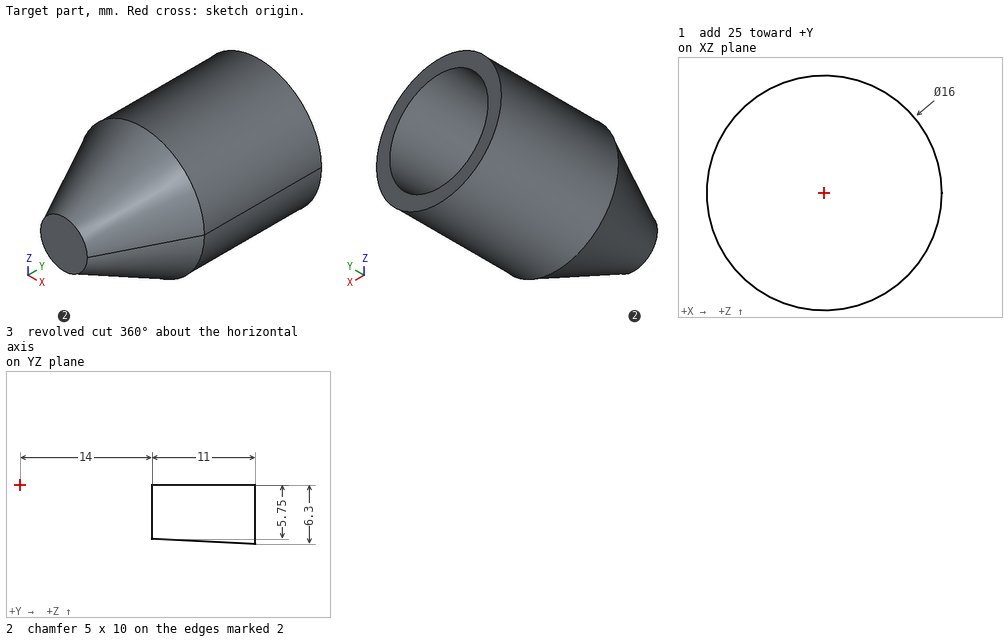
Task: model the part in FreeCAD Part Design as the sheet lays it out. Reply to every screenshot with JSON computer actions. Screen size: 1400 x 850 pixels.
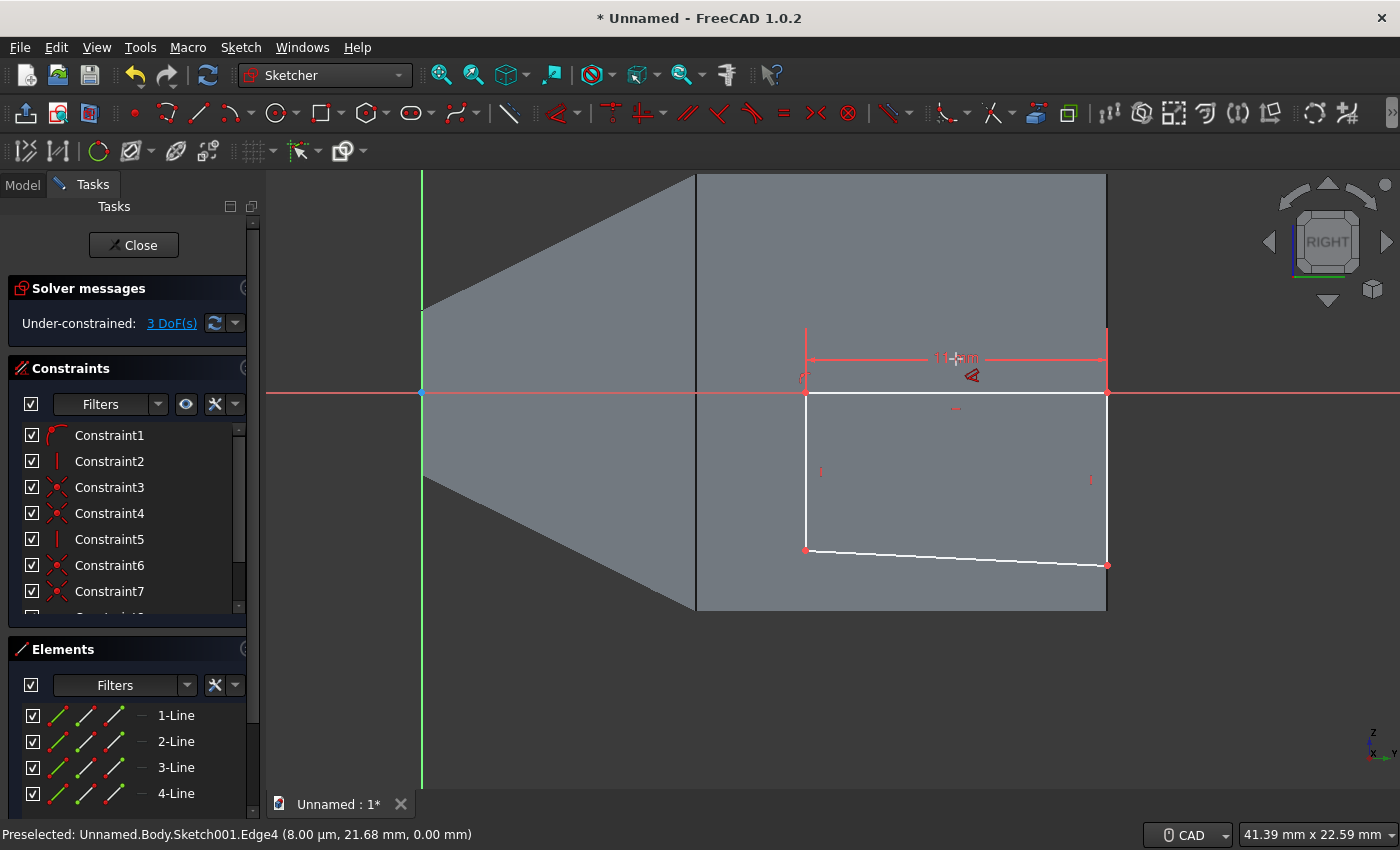
{"action": "left_click", "coordinate": [1107, 514]}
{"action": "left_click", "coordinate": [1141, 479]}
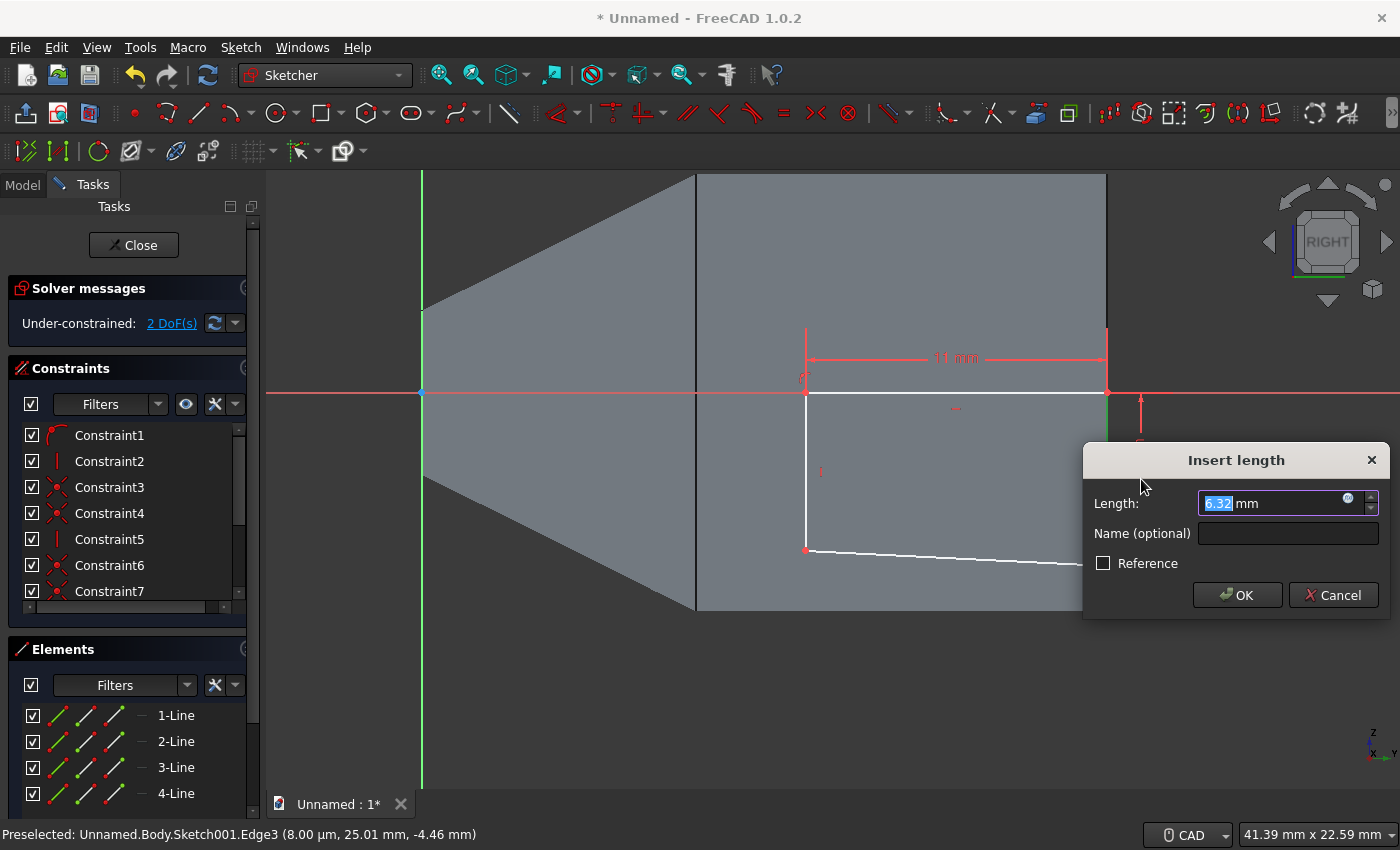
{"action": "type", "text": "6.3"}
{"action": "key", "text": "Return"}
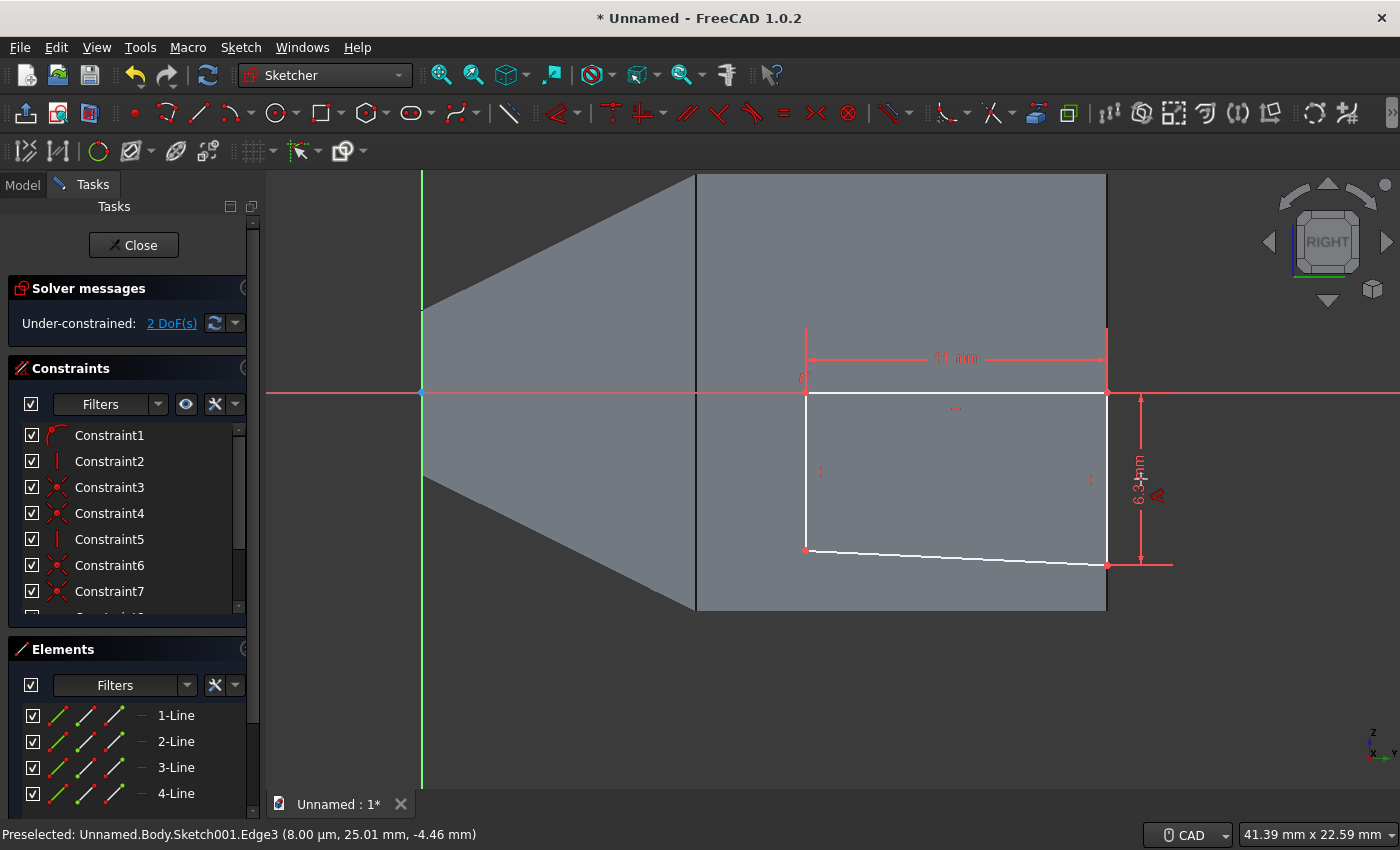
{"action": "left_click", "coordinate": [806, 393]}
{"action": "left_click", "coordinate": [614, 359]}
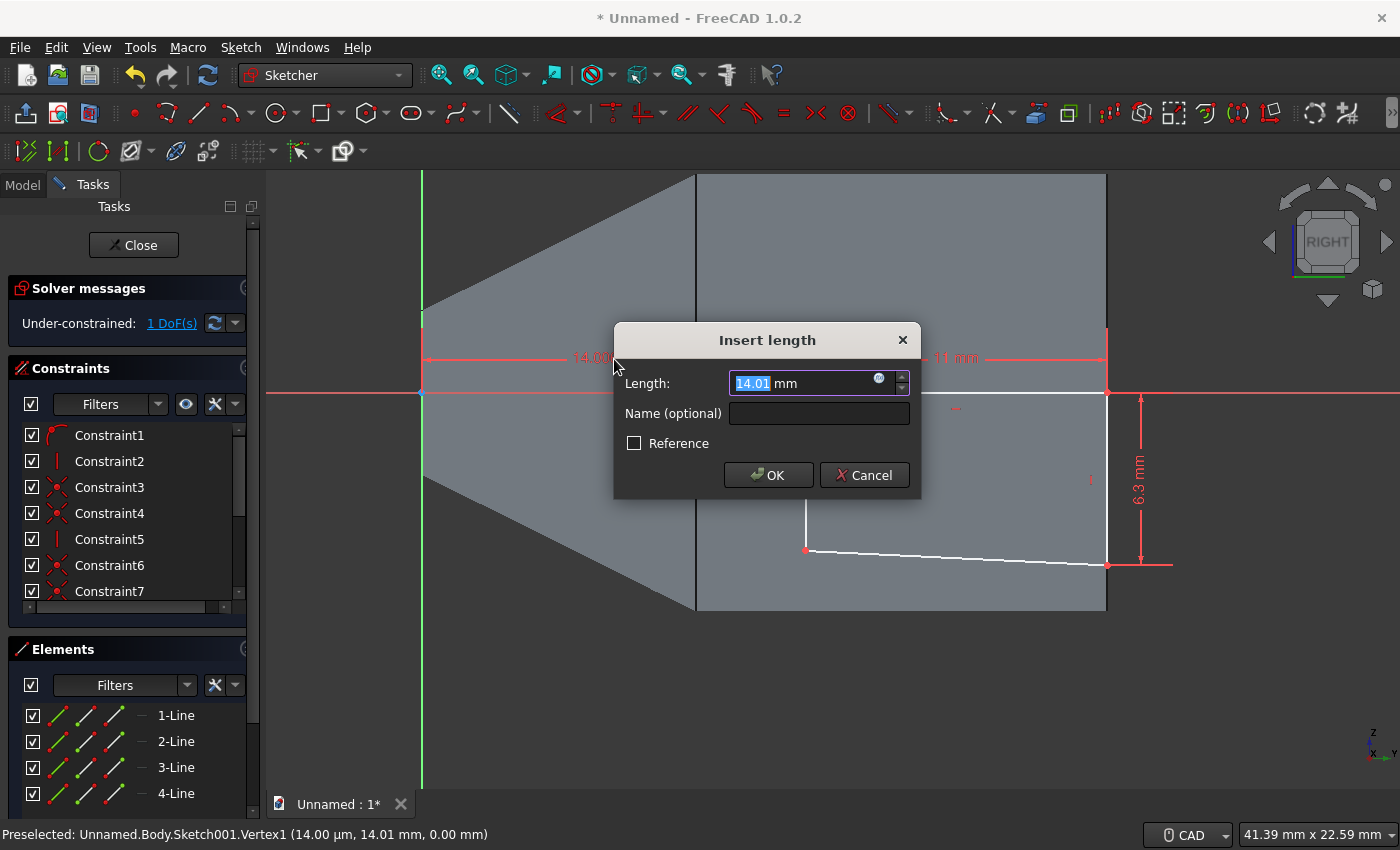
{"action": "type", "text": "14"}
{"action": "key", "text": "Return"}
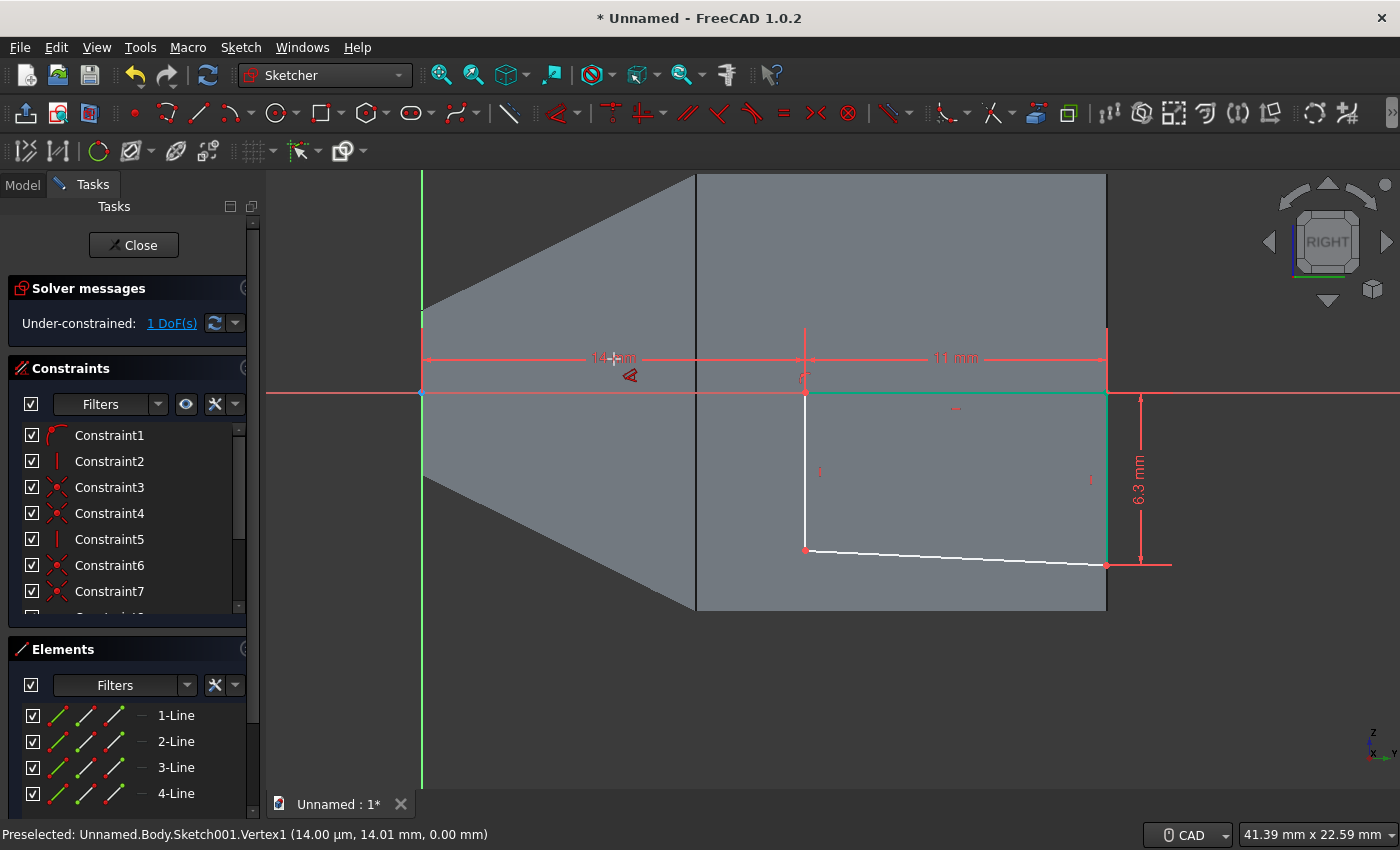
{"action": "left_click", "coordinate": [805, 440]}
{"action": "left_click", "coordinate": [839, 472]}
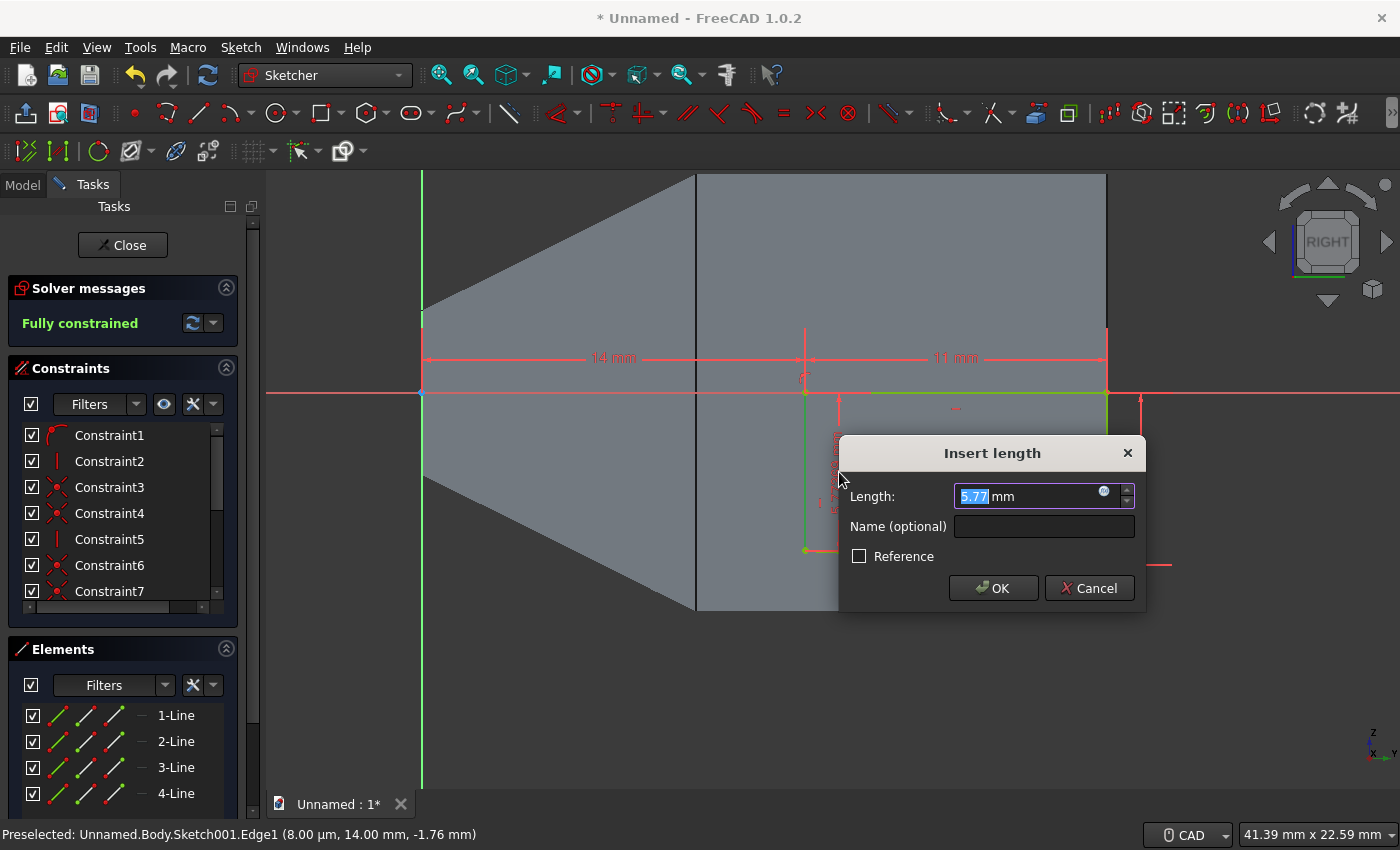
{"action": "type", "text": "5.75"}
{"action": "key", "text": "Return"}
{"action": "key", "text": "Escape"}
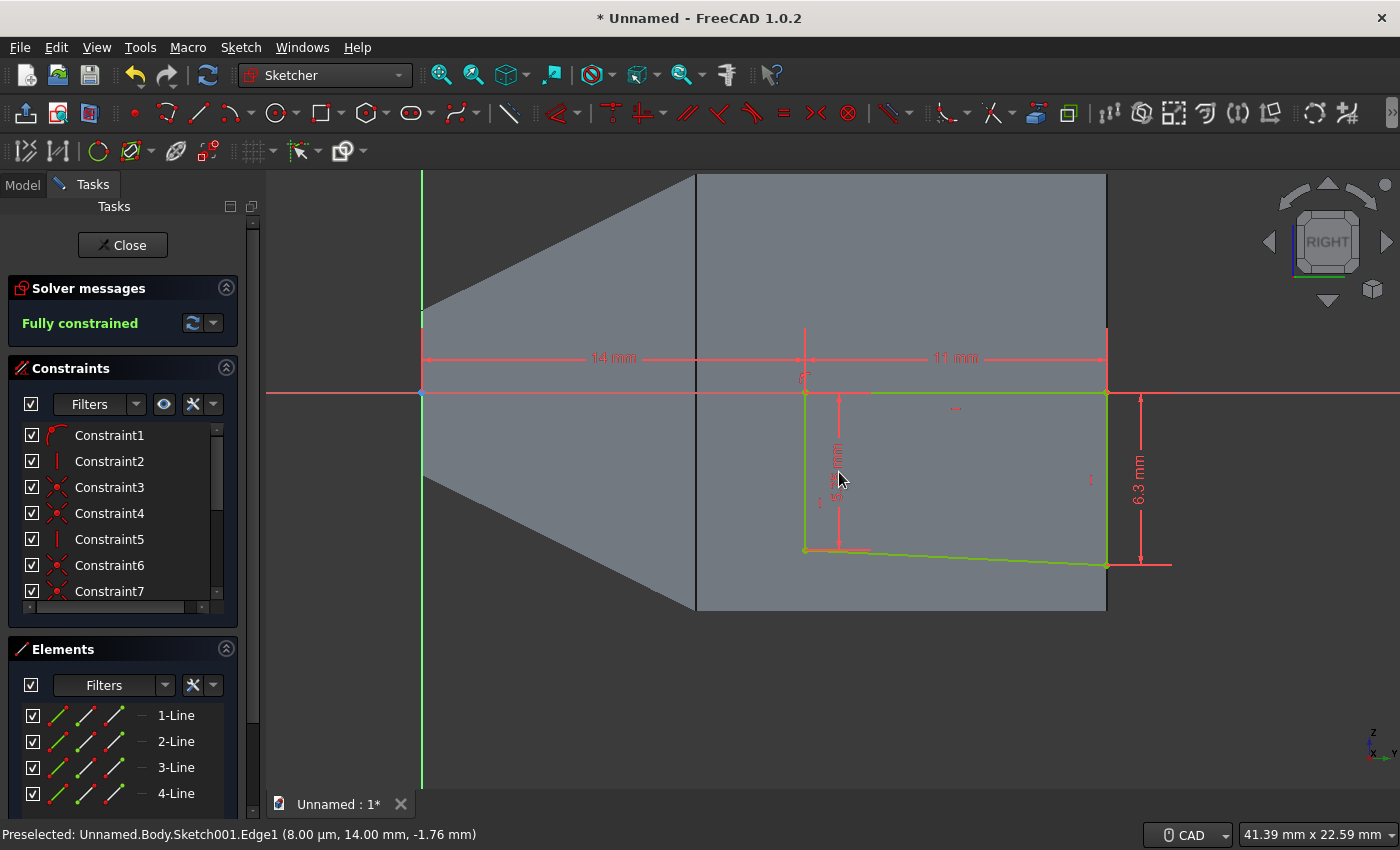
{"action": "left_click", "coordinate": [123, 245]}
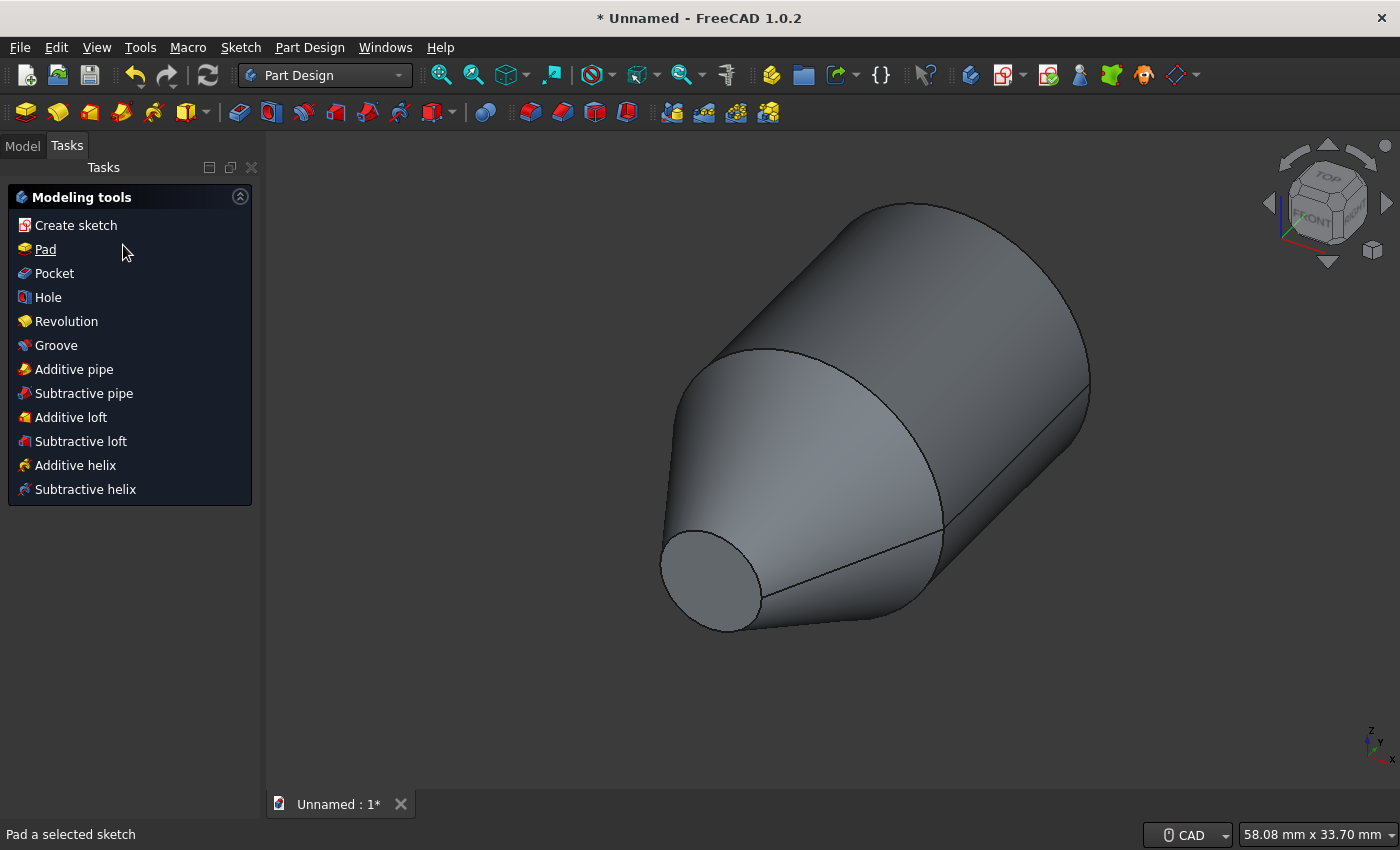
{"action": "left_click", "coordinate": [304, 112]}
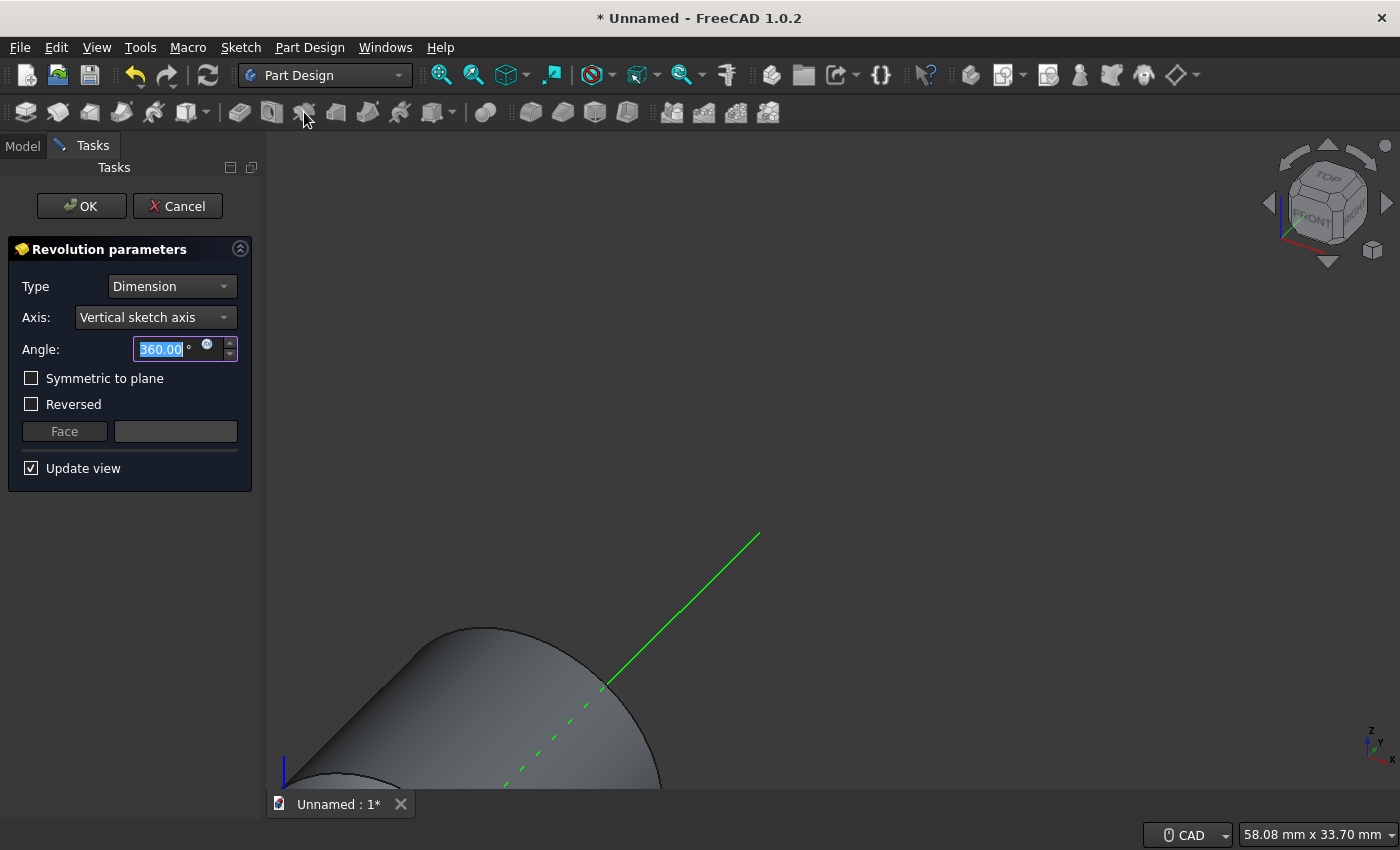
{"action": "left_click", "coordinate": [156, 318]}